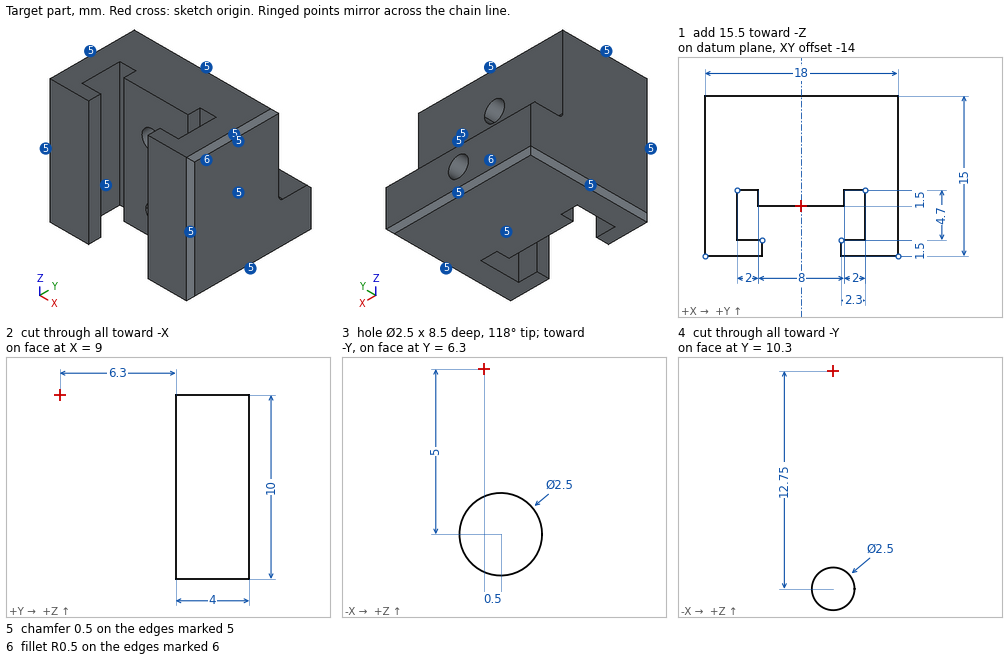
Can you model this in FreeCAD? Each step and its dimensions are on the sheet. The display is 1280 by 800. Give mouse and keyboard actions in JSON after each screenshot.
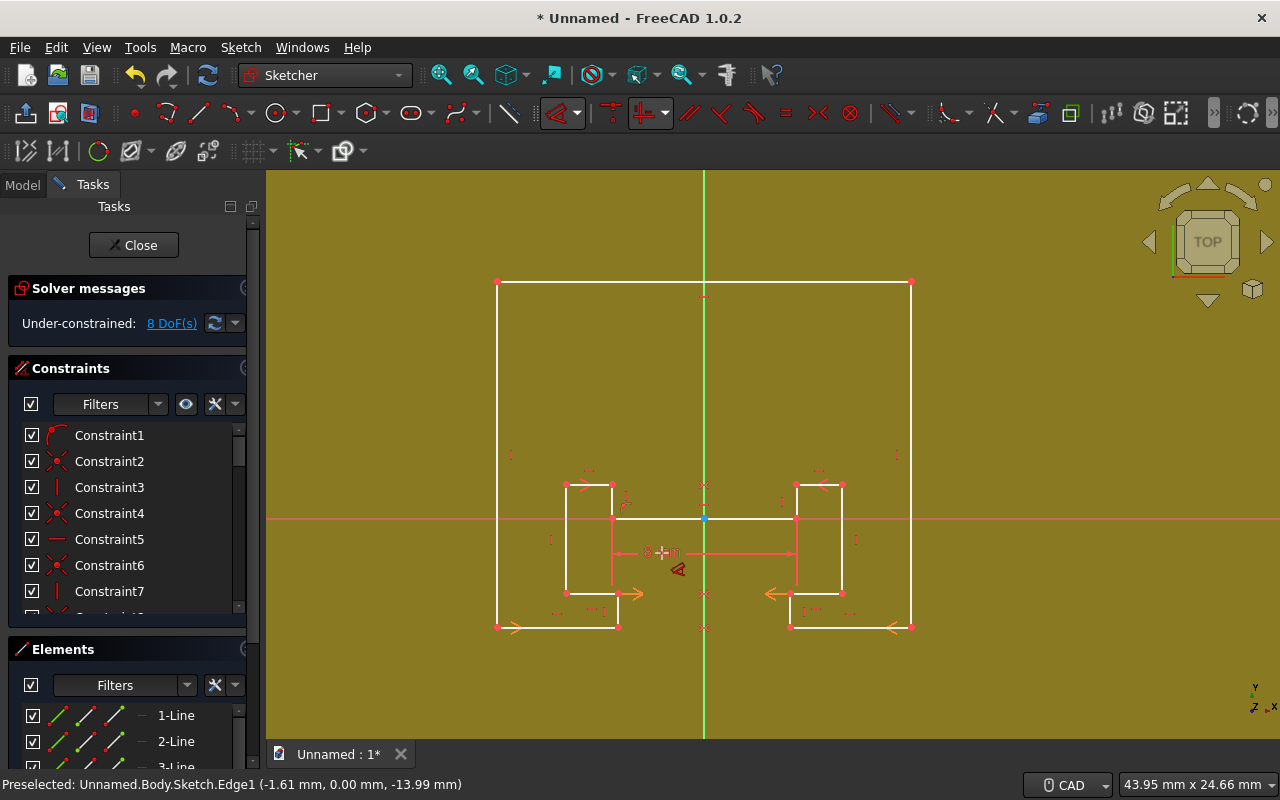
{"action": "left_click", "coordinate": [810, 485]}
{"action": "left_click", "coordinate": [819, 451]}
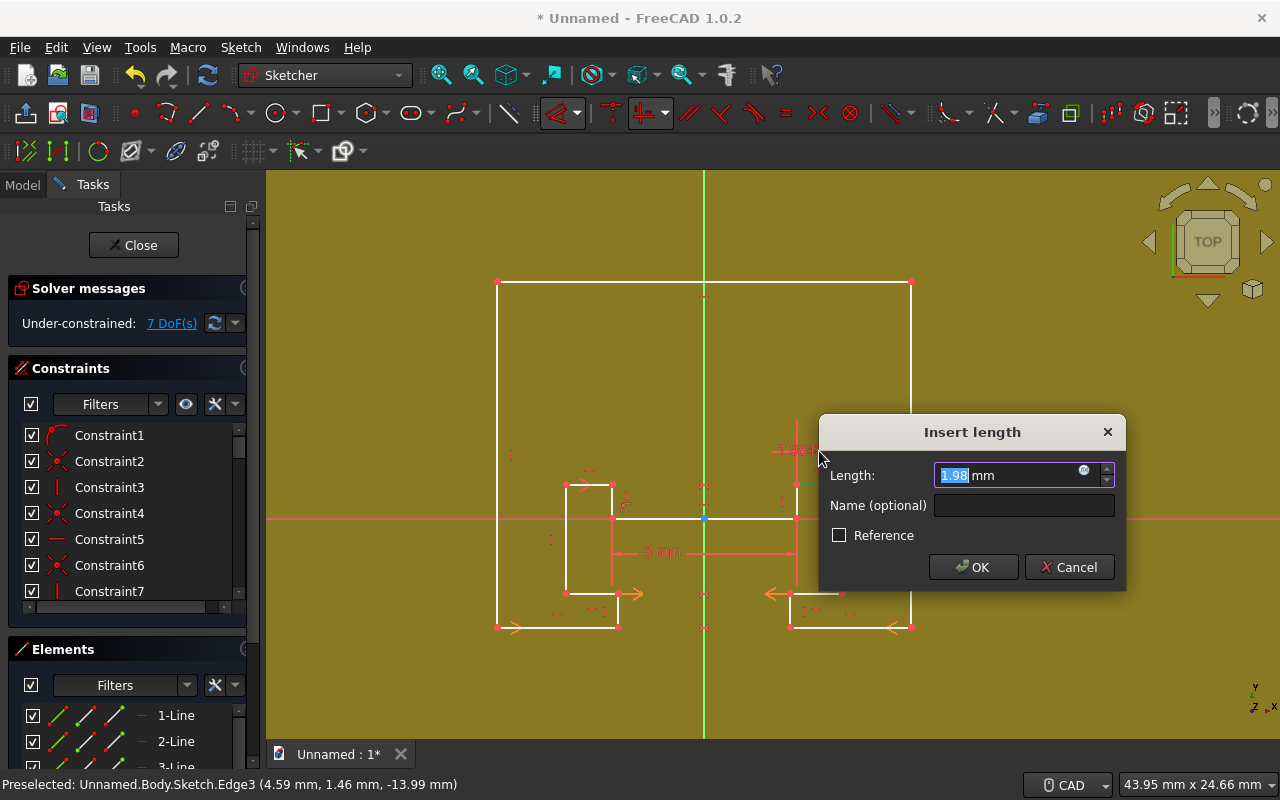
{"action": "type", "text": "2"}
{"action": "key", "text": "Return"}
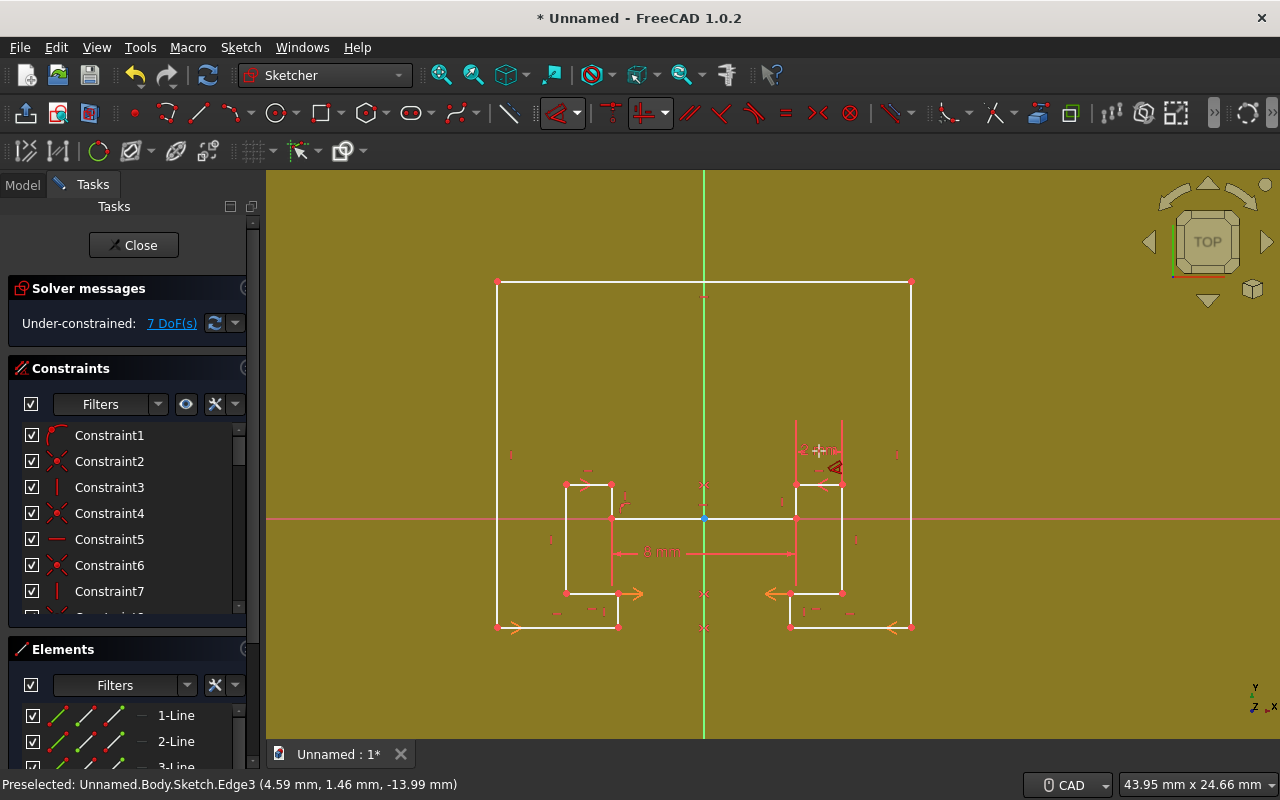
{"action": "left_click", "coordinate": [580, 485]}
{"action": "left_click", "coordinate": [589, 451]}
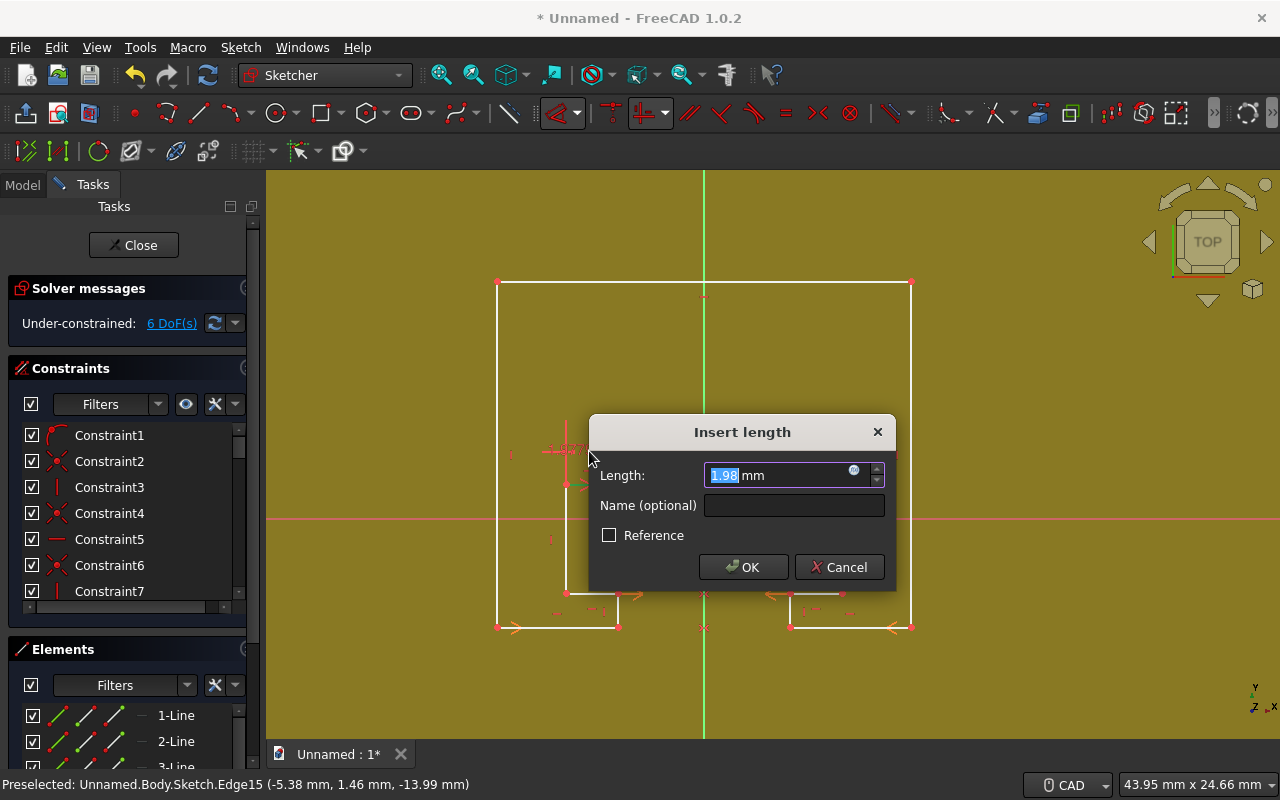
{"action": "type", "text": "2"}
{"action": "key", "text": "Return"}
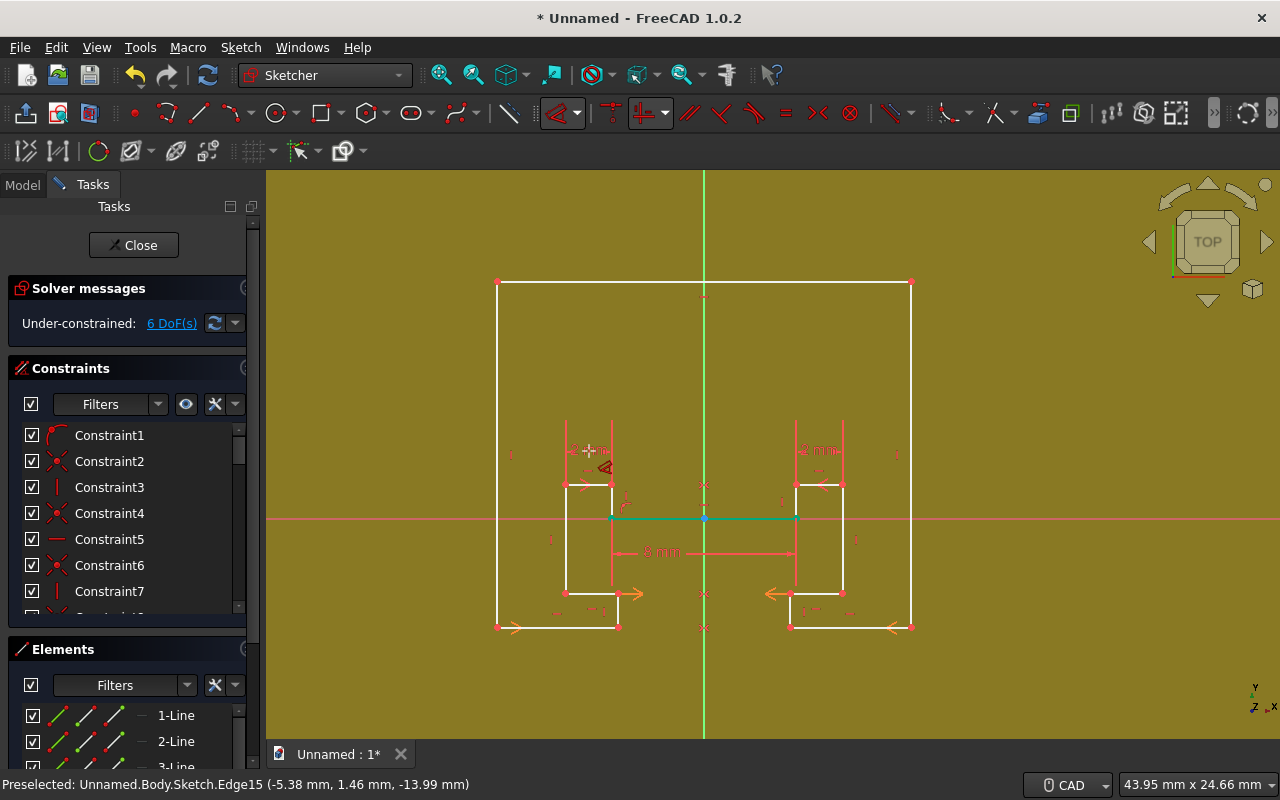
{"action": "left_click", "coordinate": [911, 386]}
{"action": "left_click", "coordinate": [945, 455]}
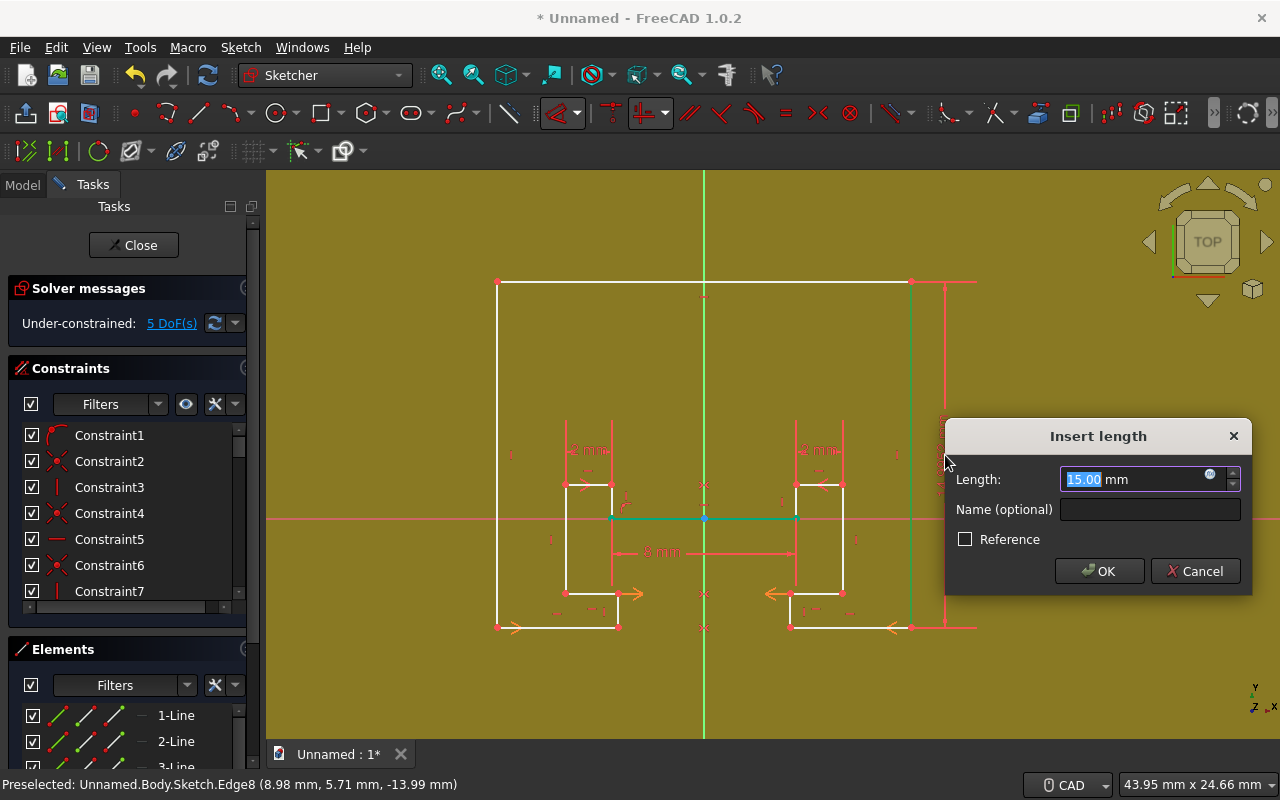
{"action": "type", "text": "15"}
{"action": "key", "text": "Return"}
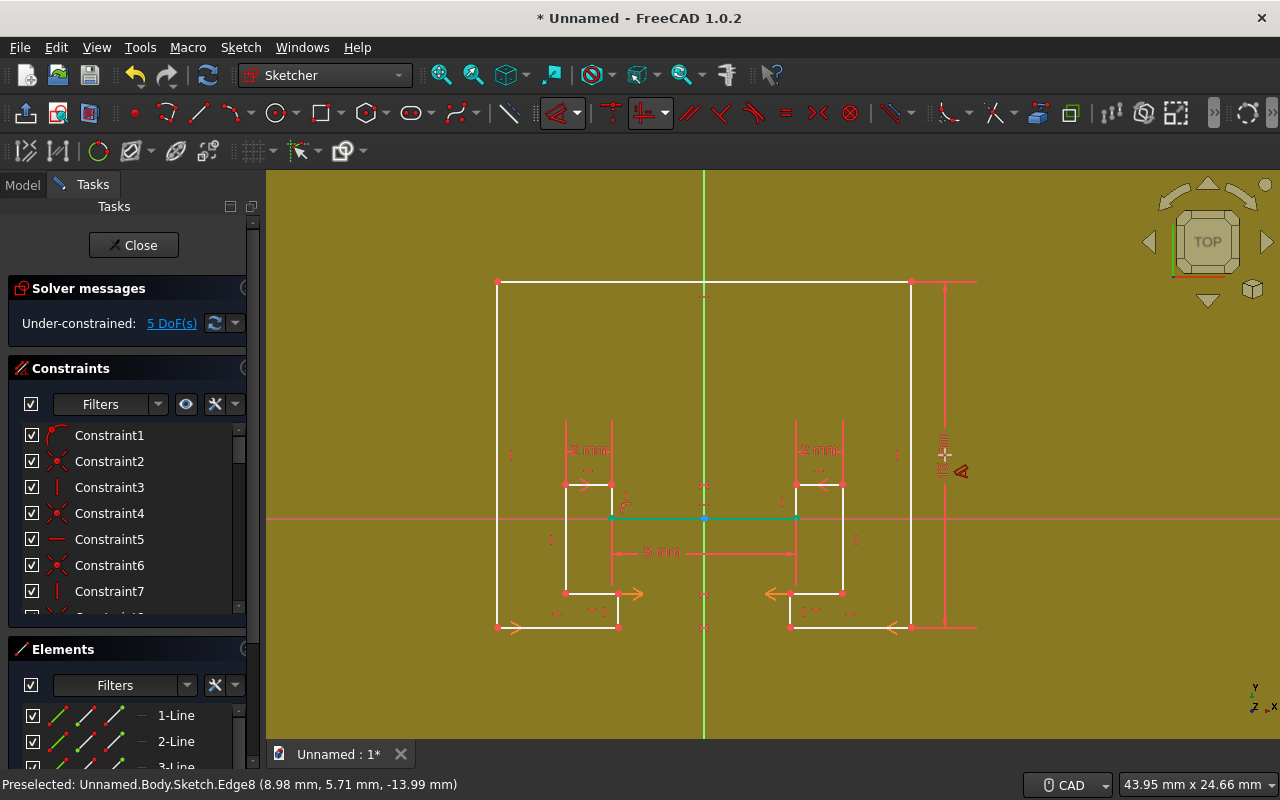
{"action": "left_click", "coordinate": [787, 282]}
{"action": "left_click", "coordinate": [609, 248]}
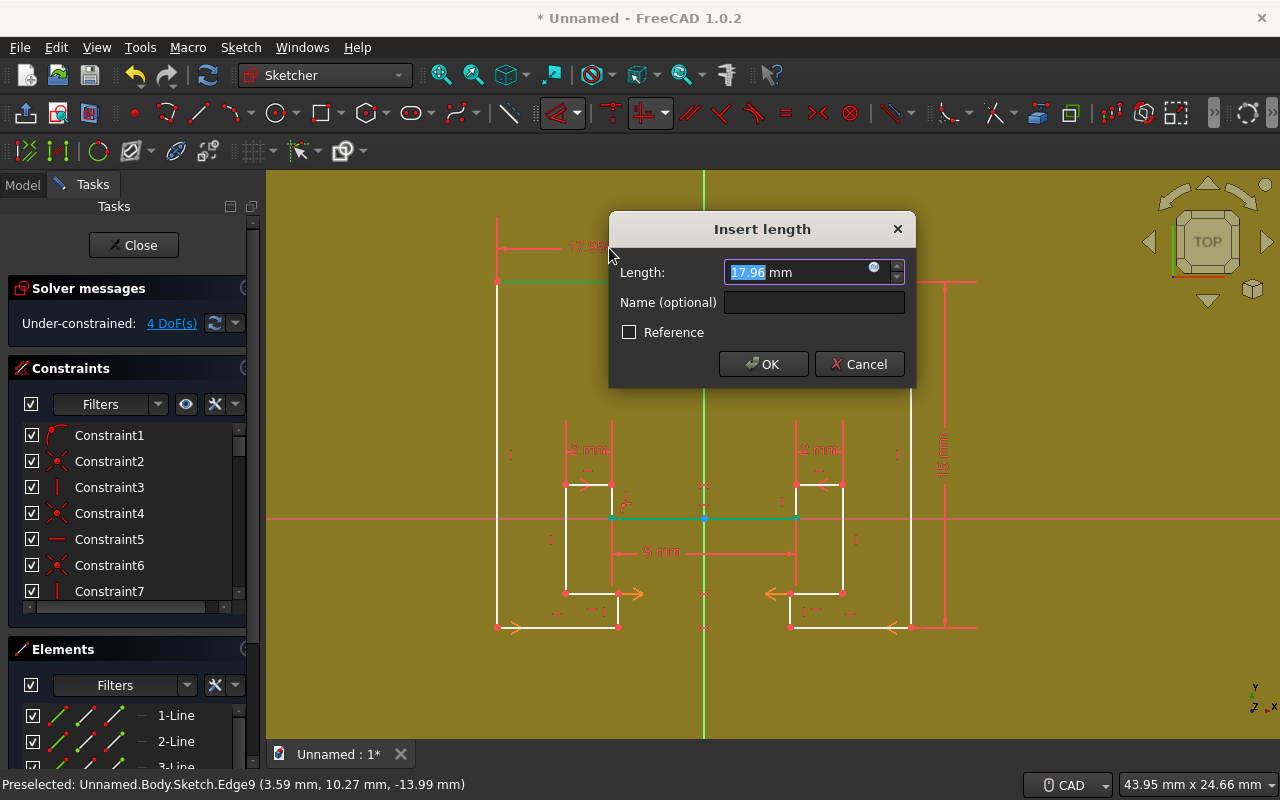
{"action": "type", "text": "18"}
{"action": "key", "text": "Return"}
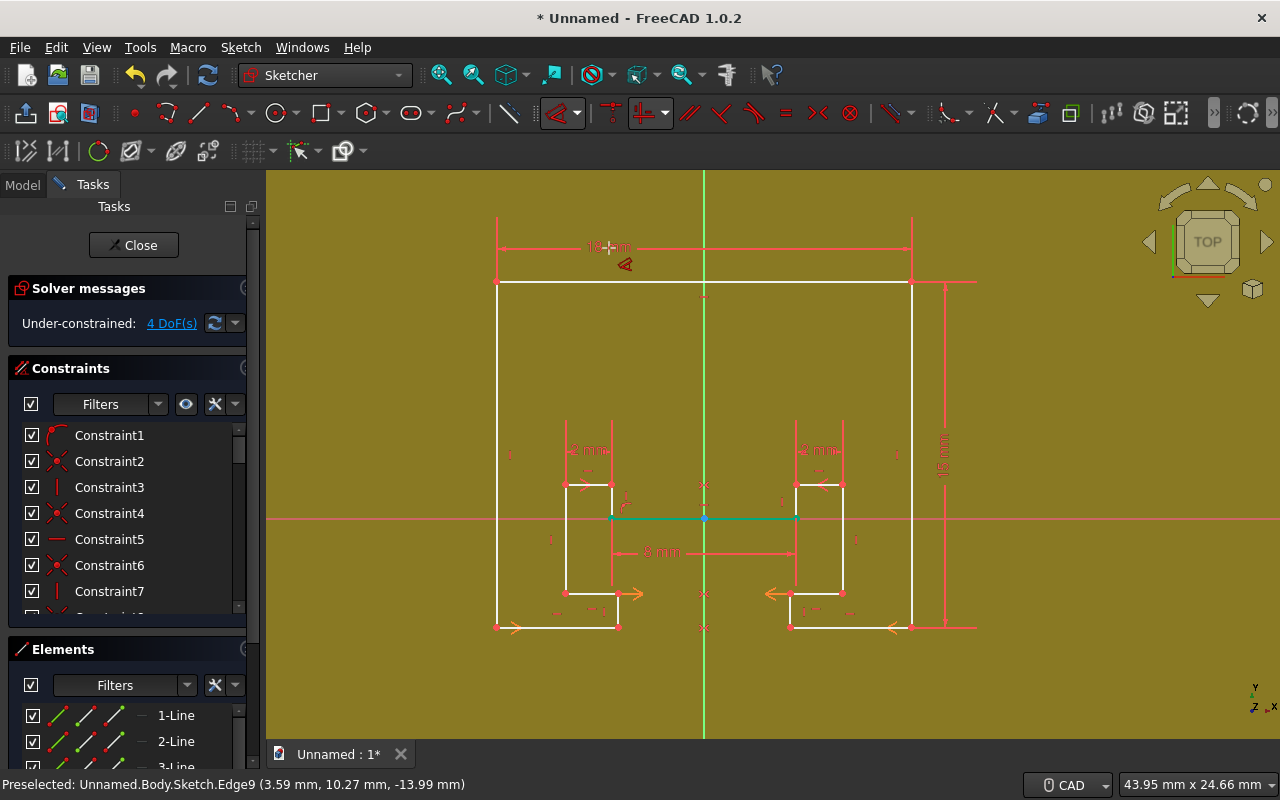
{"action": "scroll", "coordinate": [796, 509], "scroll_direction": "up", "scroll_amount": 2}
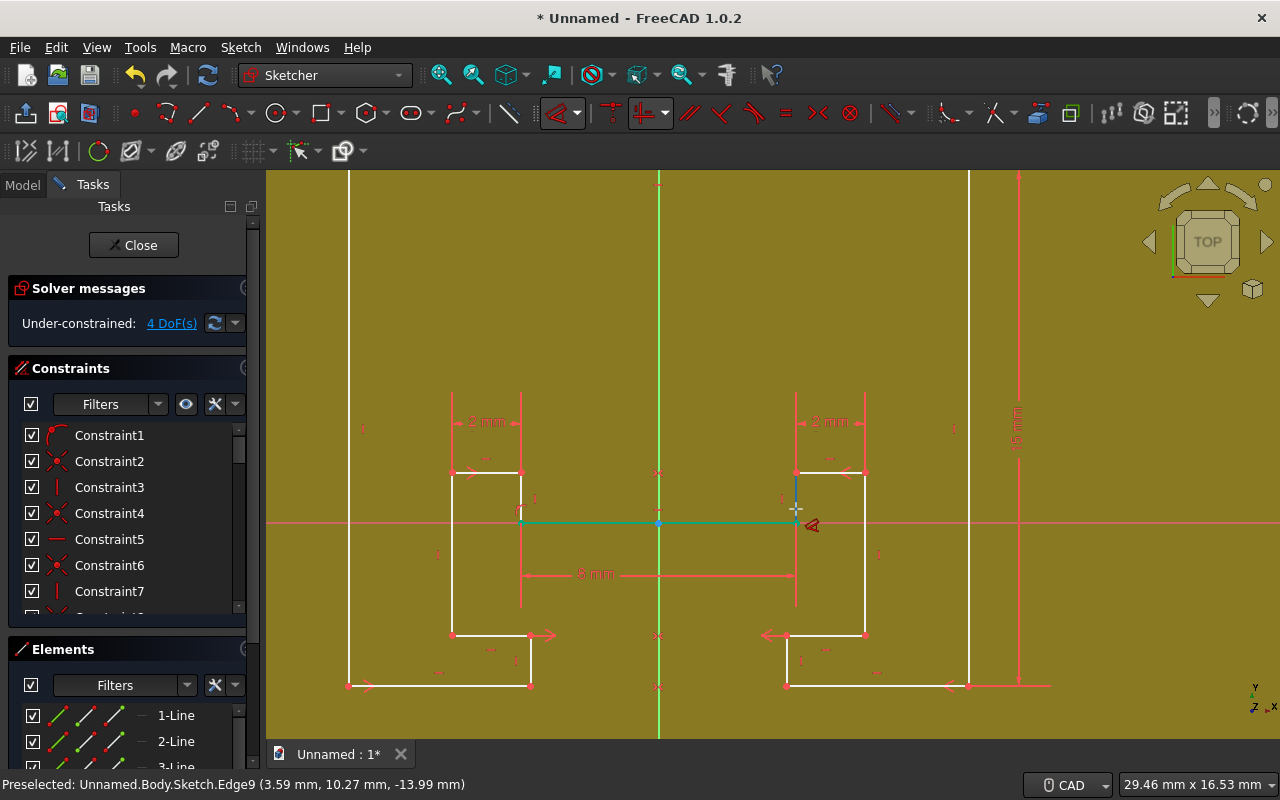
{"action": "left_click", "coordinate": [796, 508]}
{"action": "left_click", "coordinate": [830, 498]}